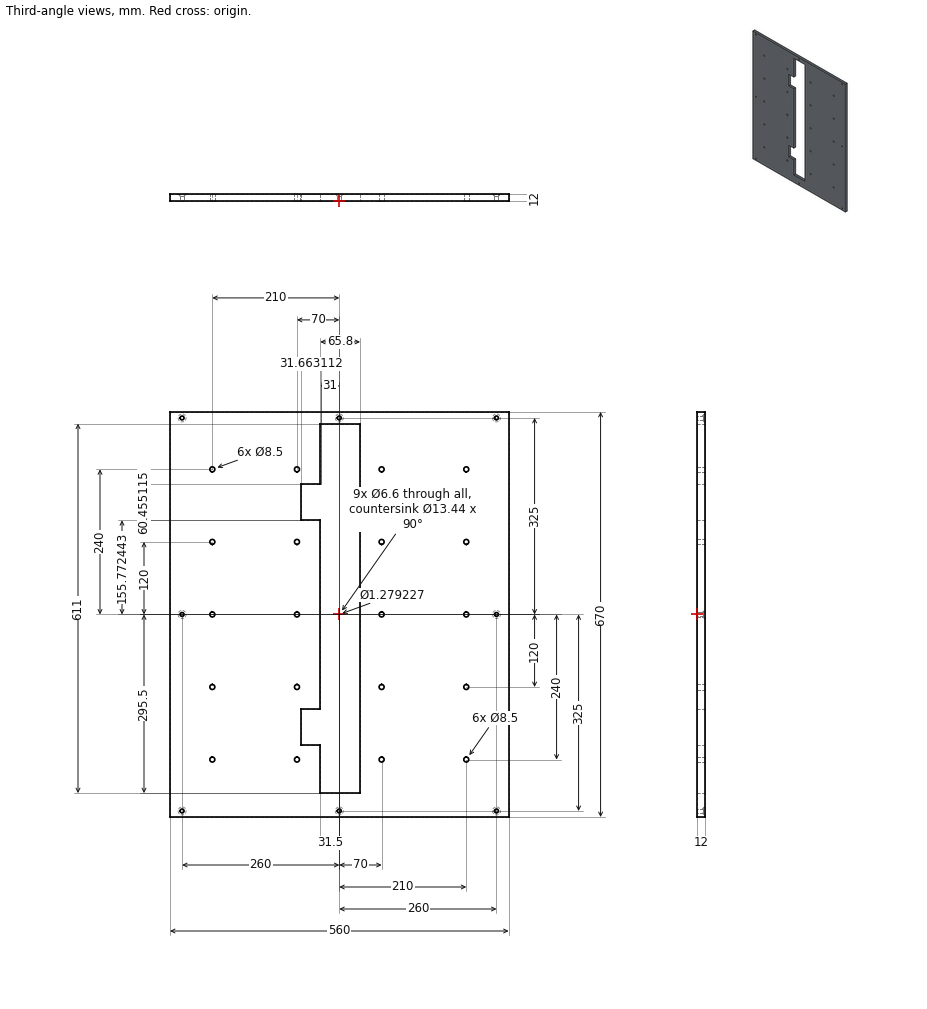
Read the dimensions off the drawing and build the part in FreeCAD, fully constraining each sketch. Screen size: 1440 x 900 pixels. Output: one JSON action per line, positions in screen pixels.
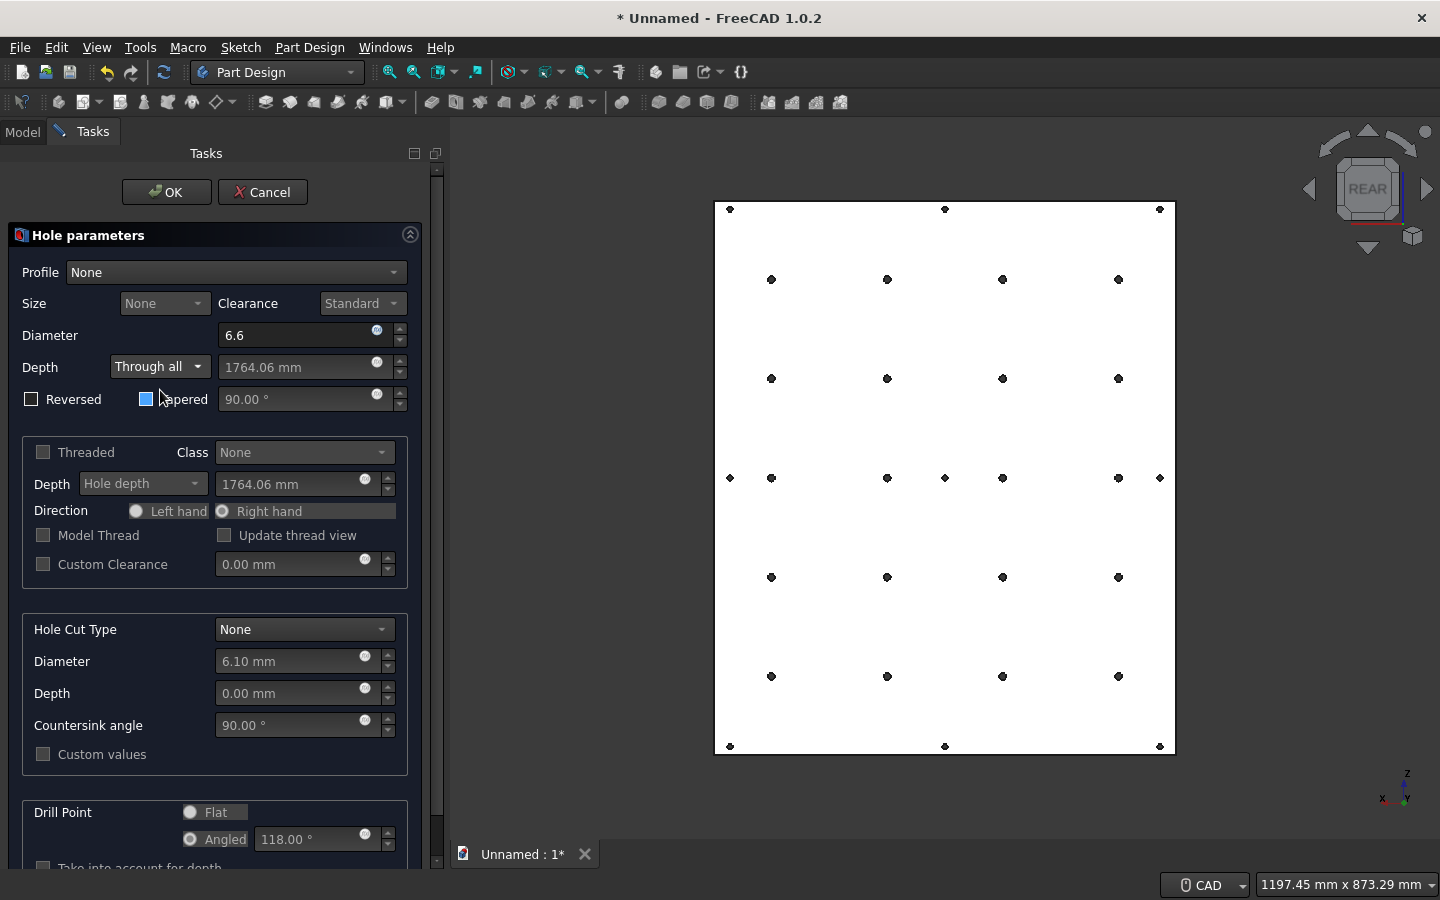
{"action": "left_click", "coordinate": [306, 630]}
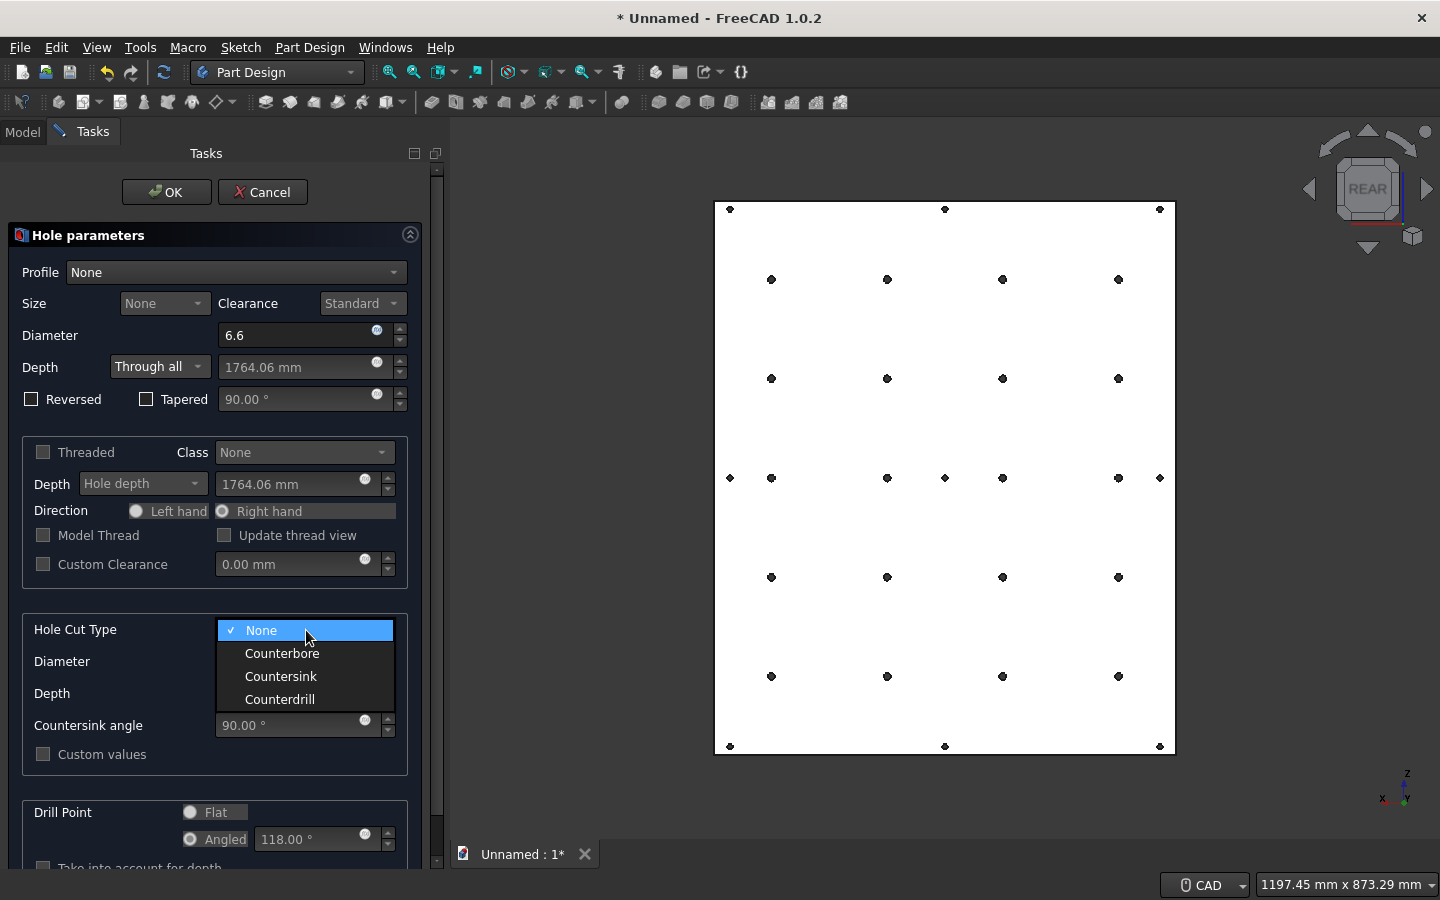
{"action": "left_click", "coordinate": [304, 676]}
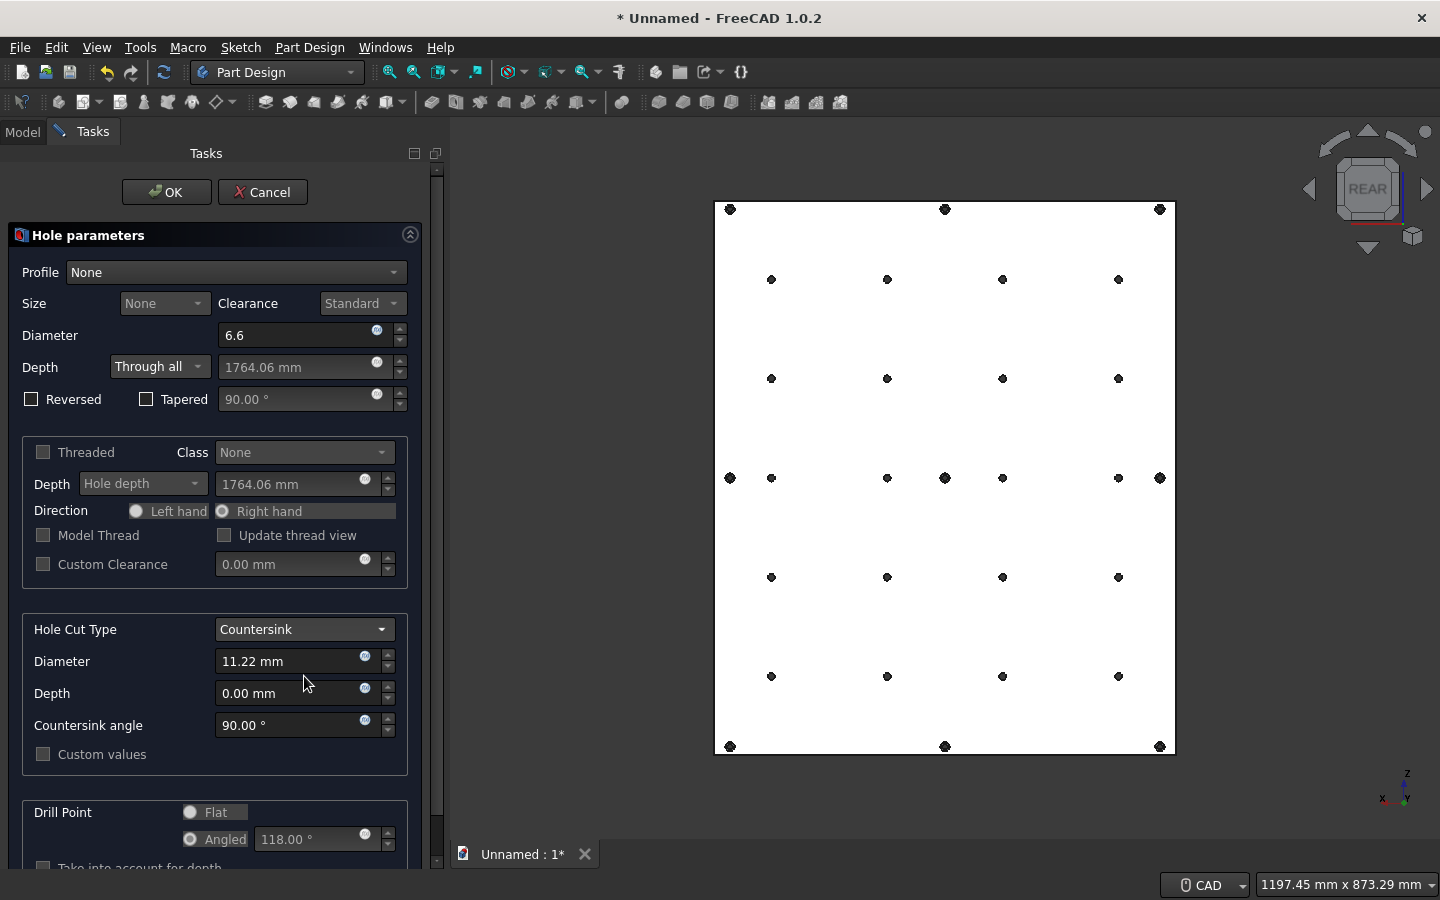
{"action": "triple_click", "coordinate": [298, 661]}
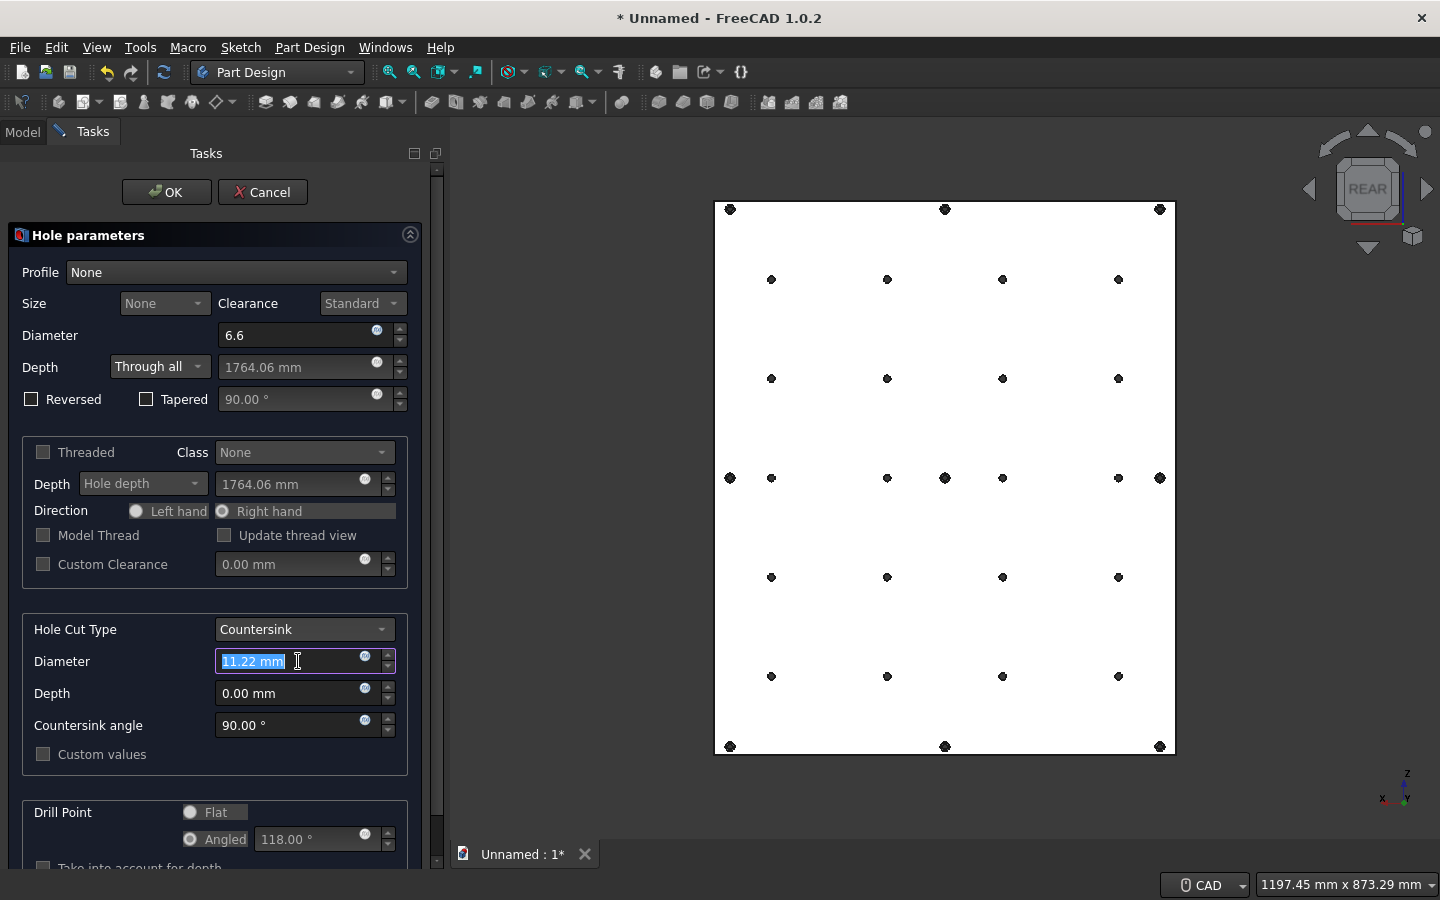
{"action": "type", "text": "13.44"}
{"action": "key", "text": "Tab"}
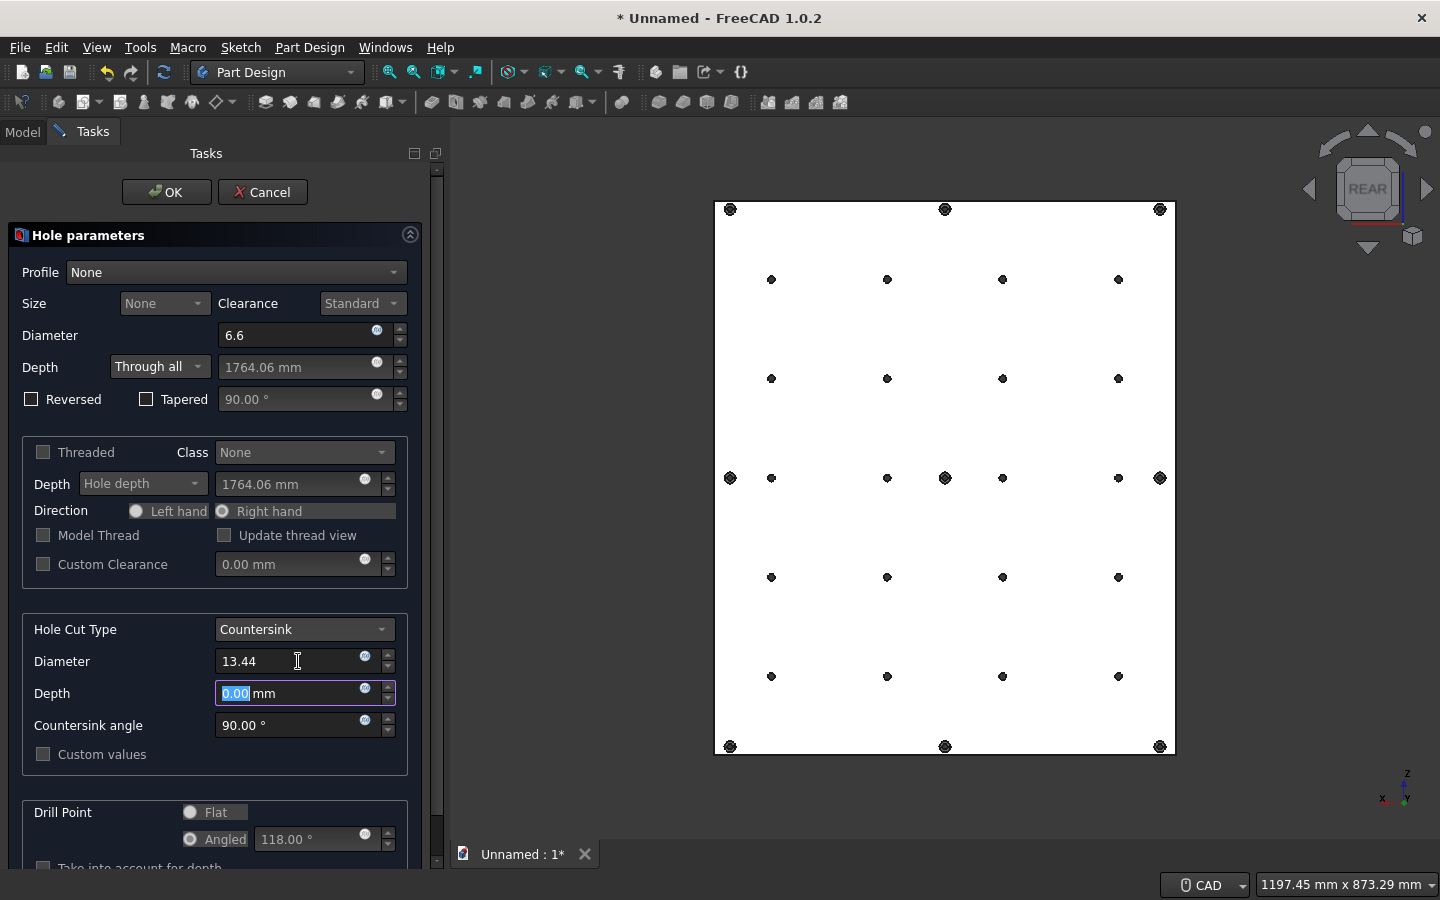
{"action": "left_click", "coordinate": [167, 192]}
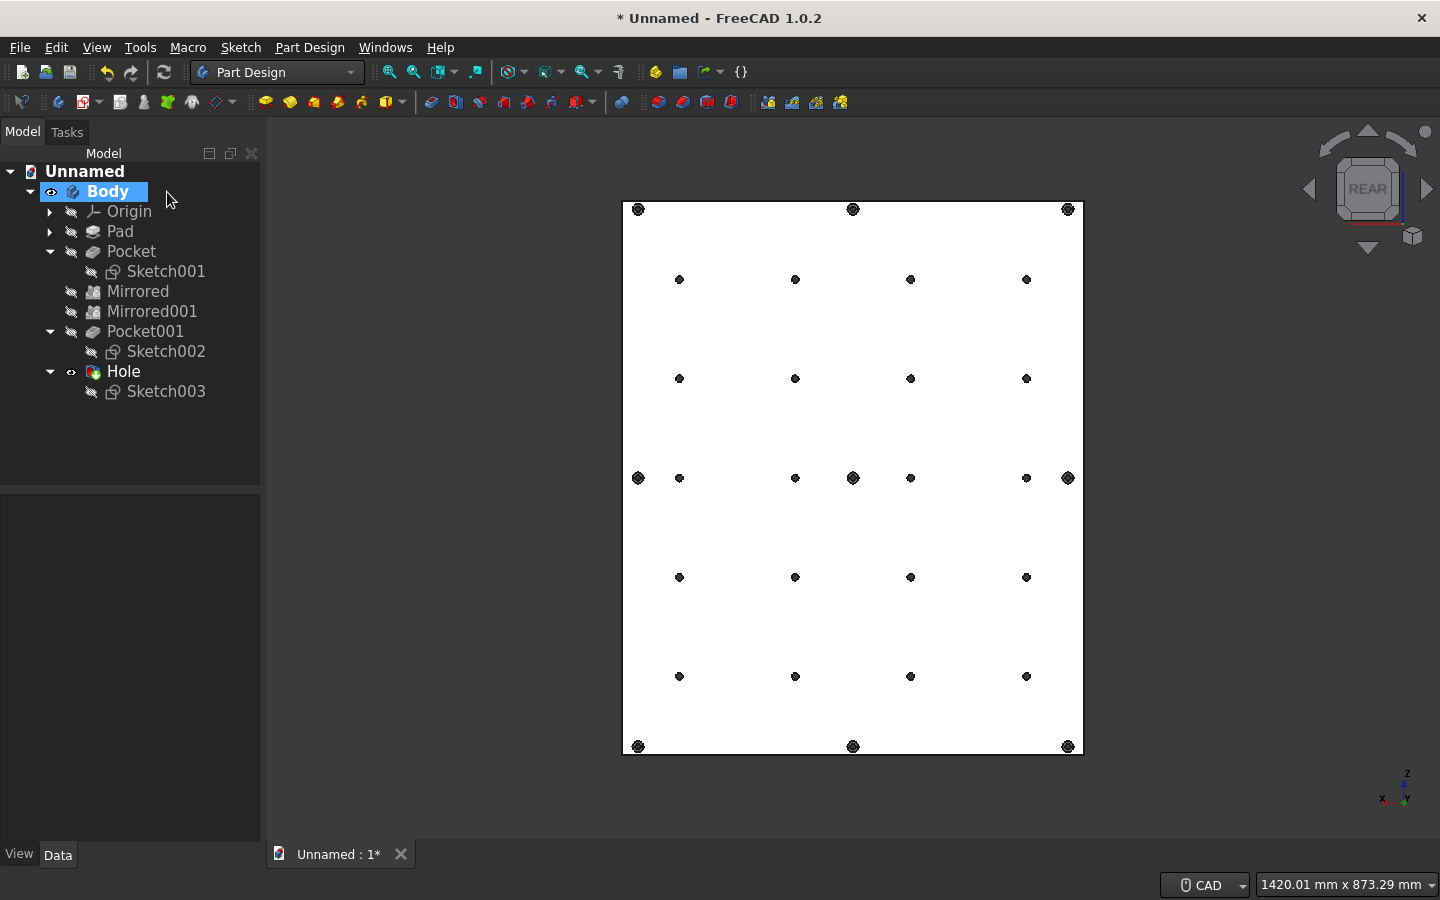
{"action": "left_click", "coordinate": [853, 635]}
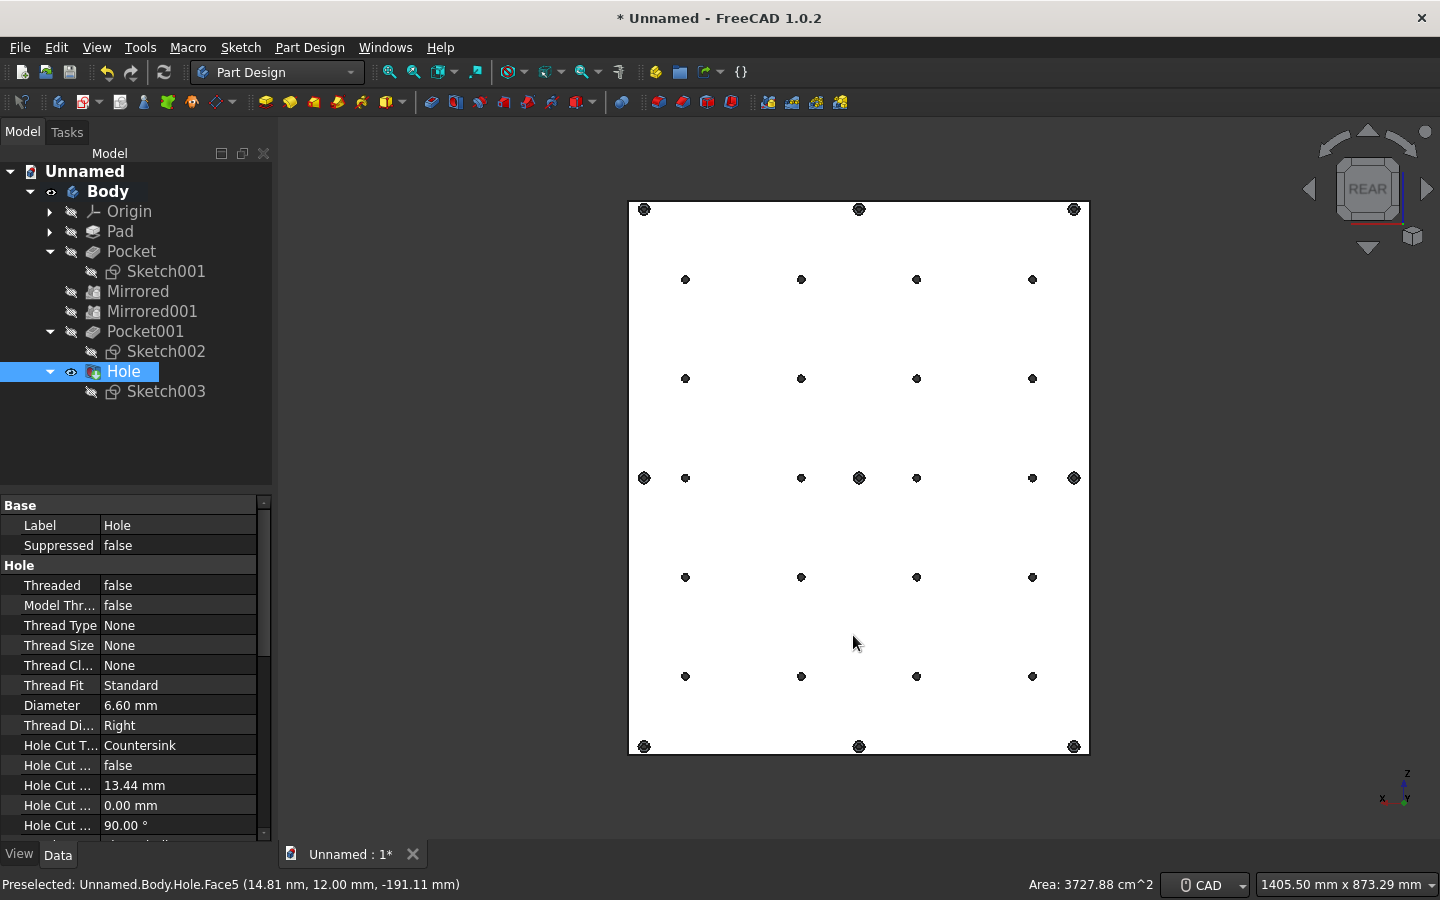
{"action": "left_click", "coordinate": [84, 102]}